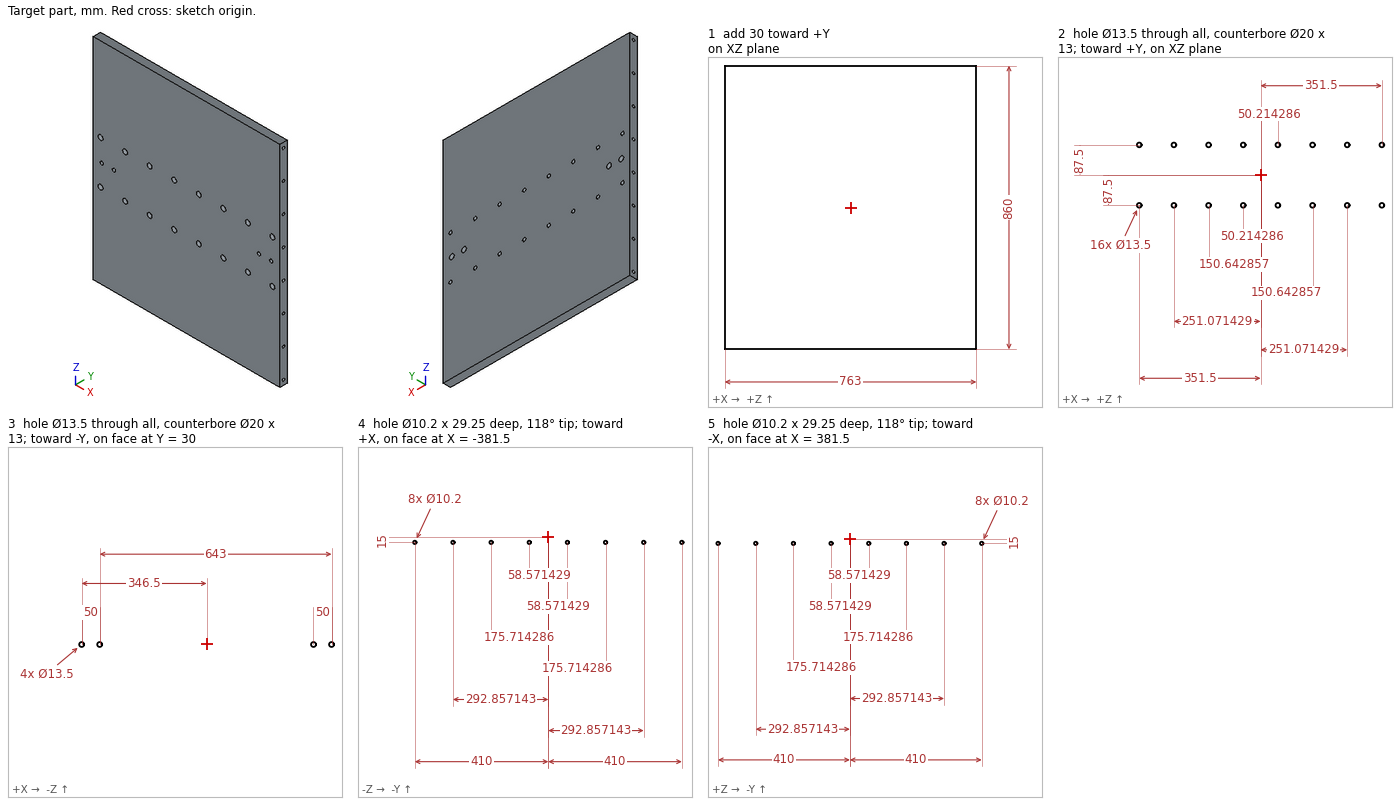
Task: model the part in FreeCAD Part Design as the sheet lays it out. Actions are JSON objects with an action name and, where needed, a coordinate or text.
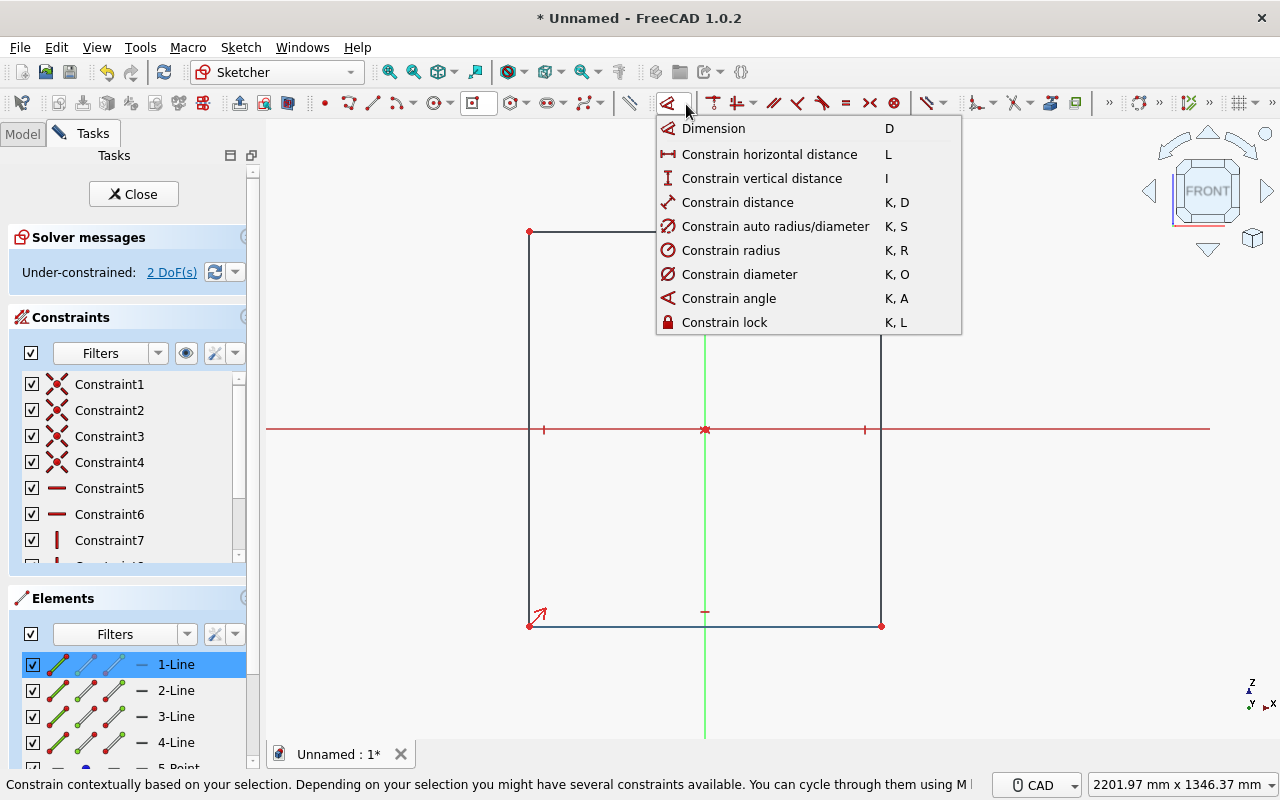
{"action": "left_click", "coordinate": [809, 154]}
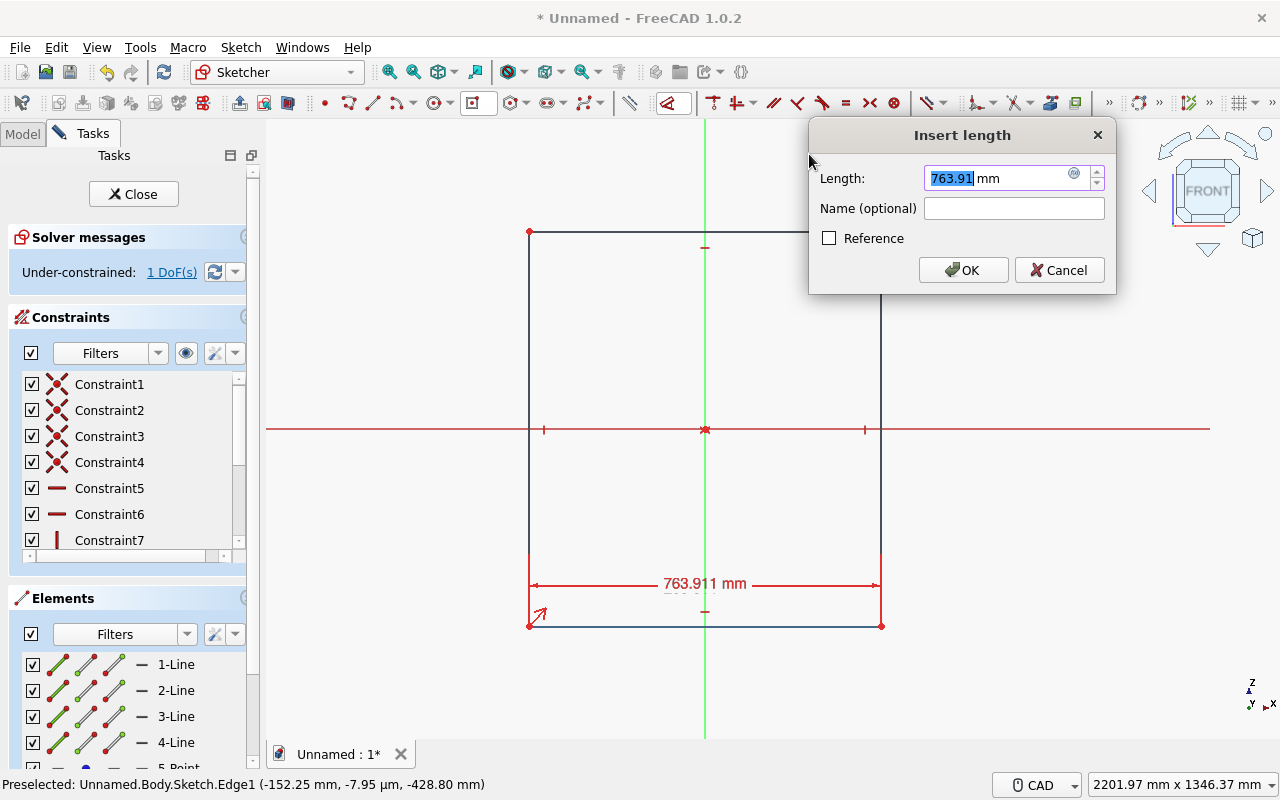
{"action": "type", "text": "763"}
{"action": "key", "text": "Return"}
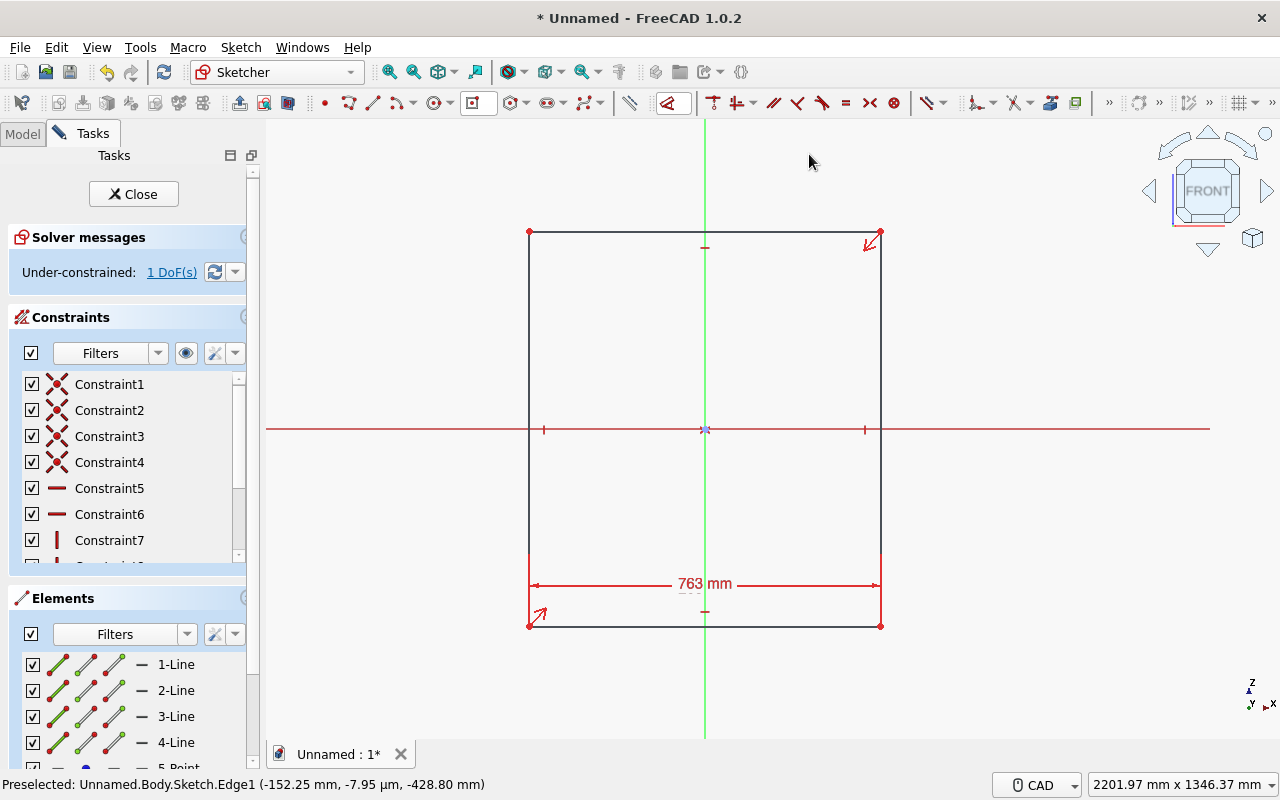
{"action": "left_click", "coordinate": [881, 508]}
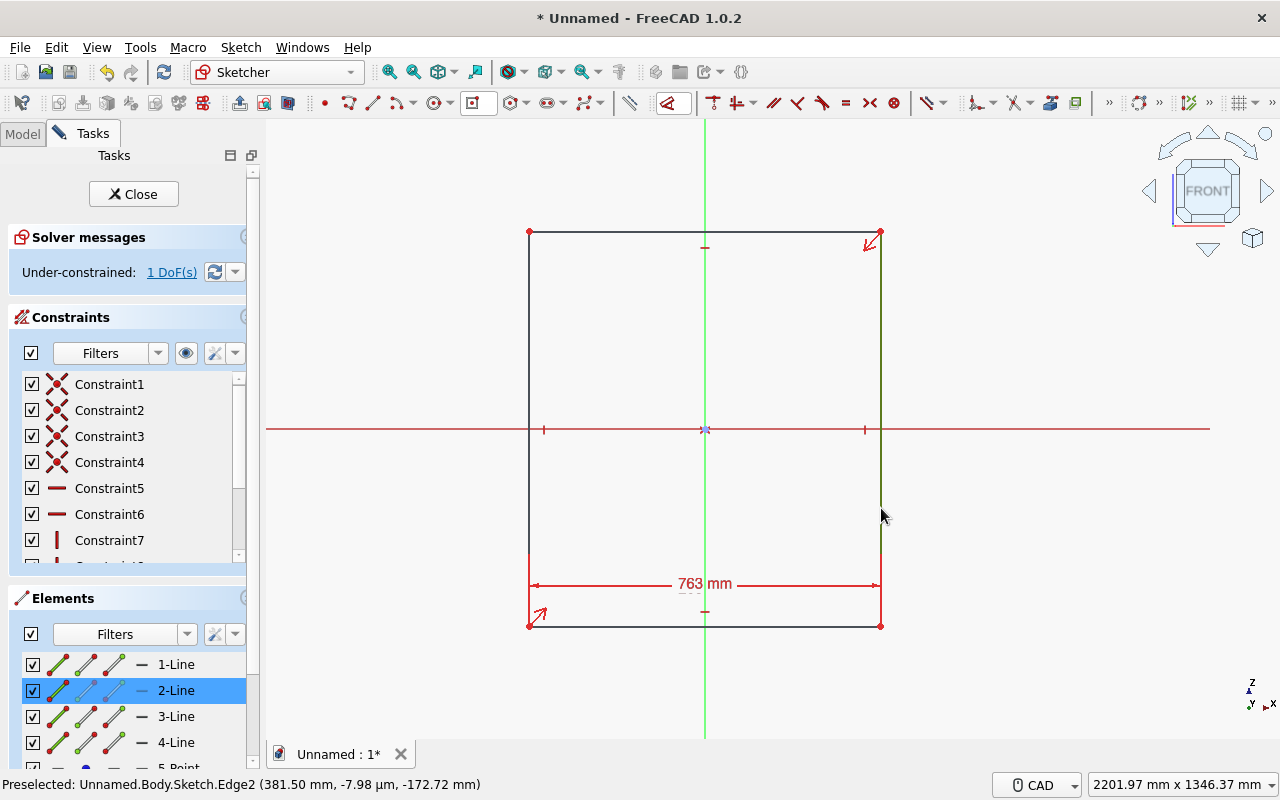
{"action": "left_click", "coordinate": [686, 104]}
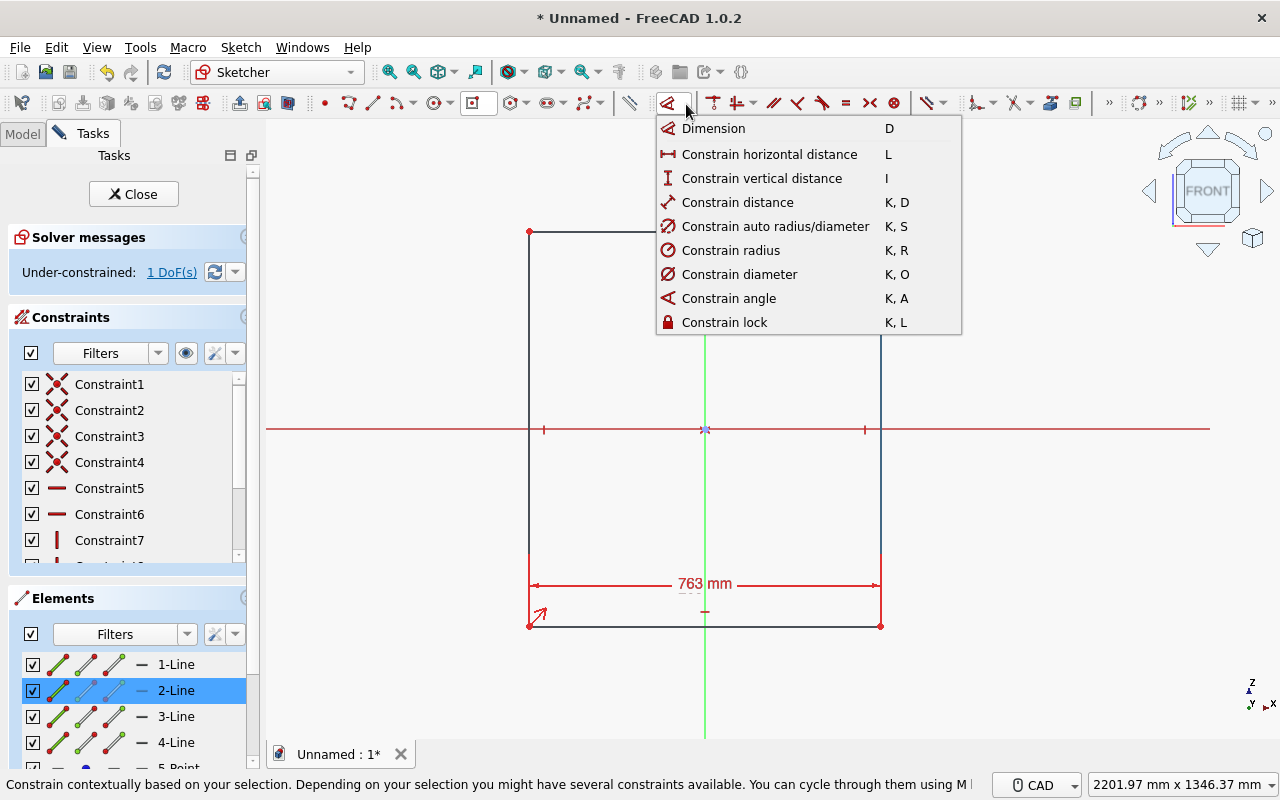
{"action": "left_click", "coordinate": [809, 178]}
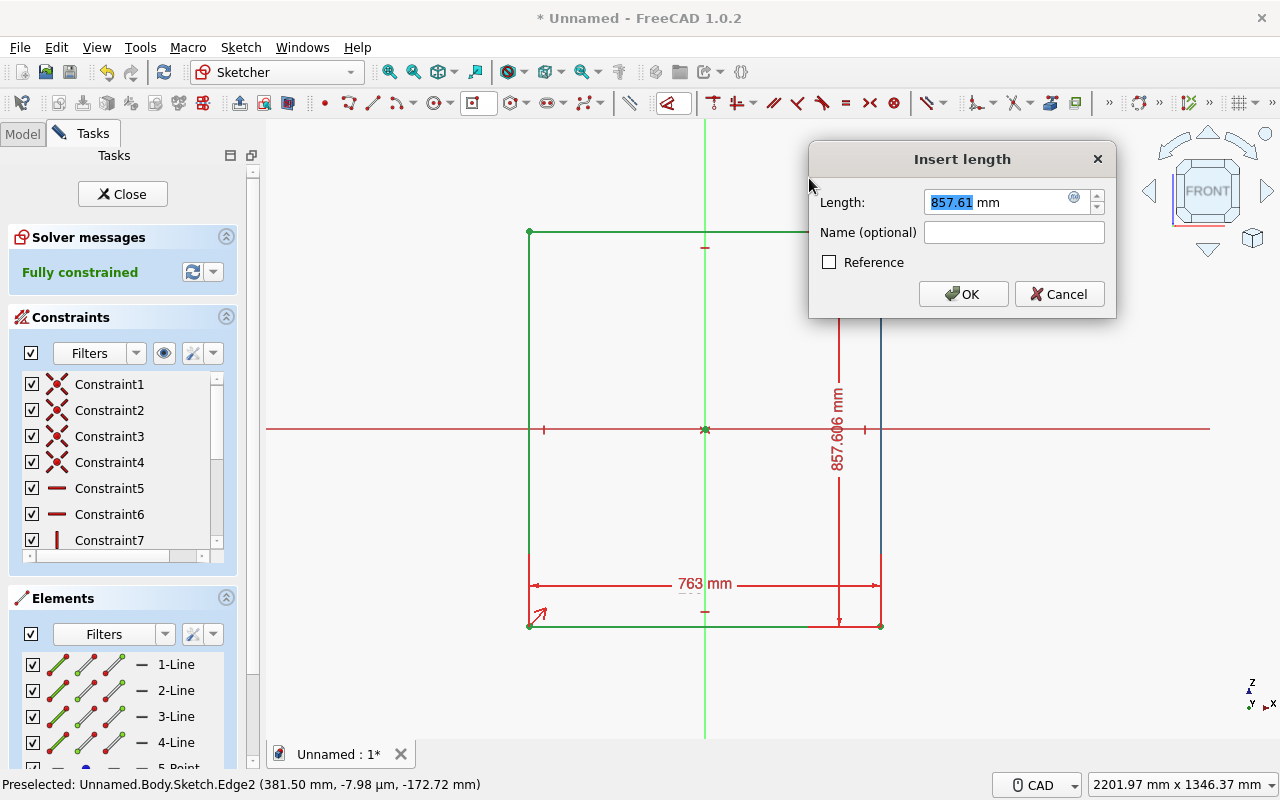
{"action": "type", "text": "860"}
{"action": "key", "text": "Return"}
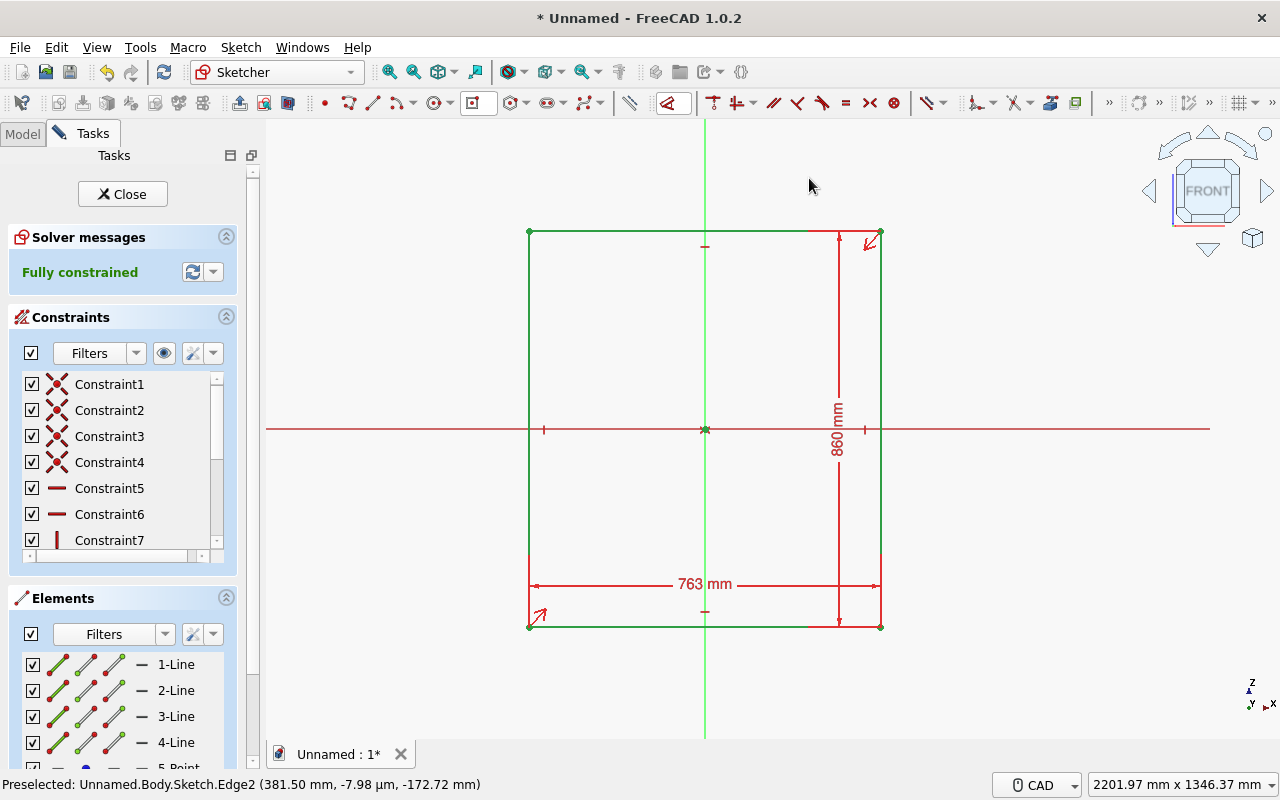
{"action": "left_click", "coordinate": [123, 194]}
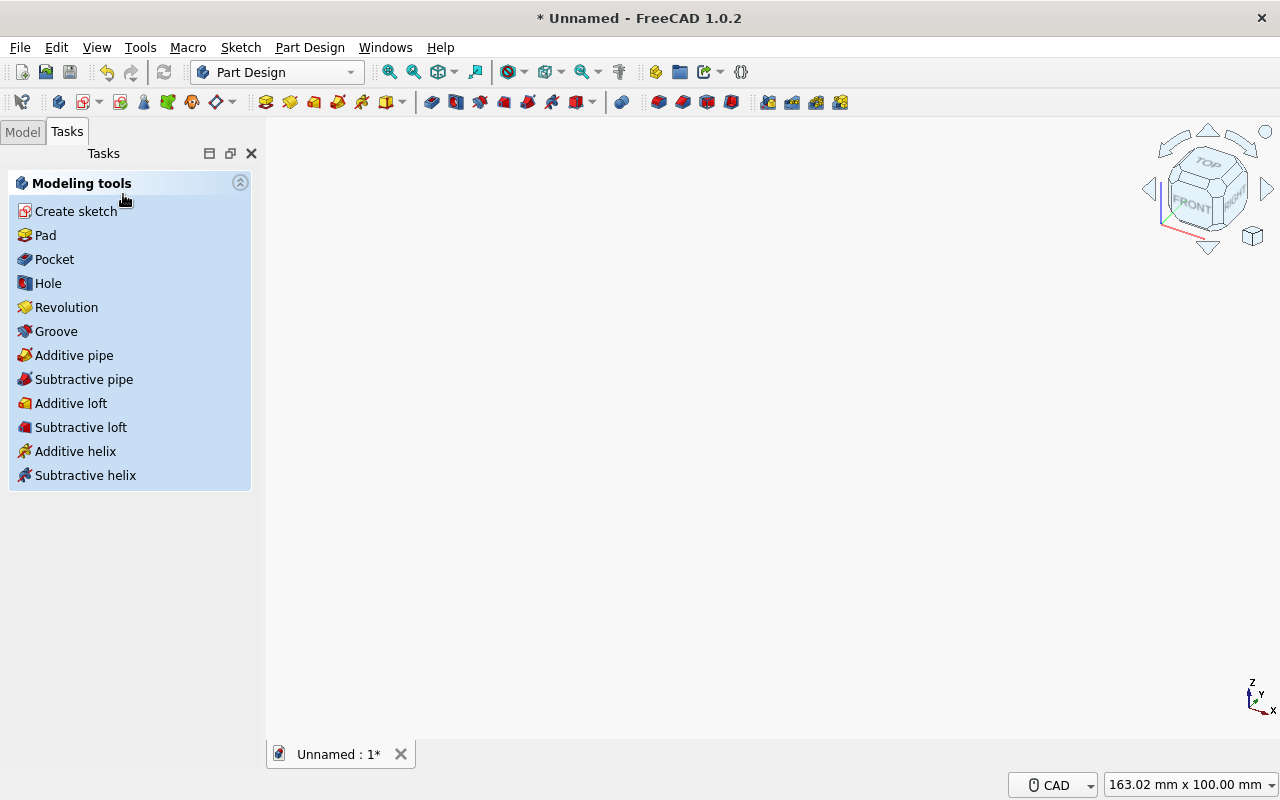
{"action": "left_click", "coordinate": [266, 102]}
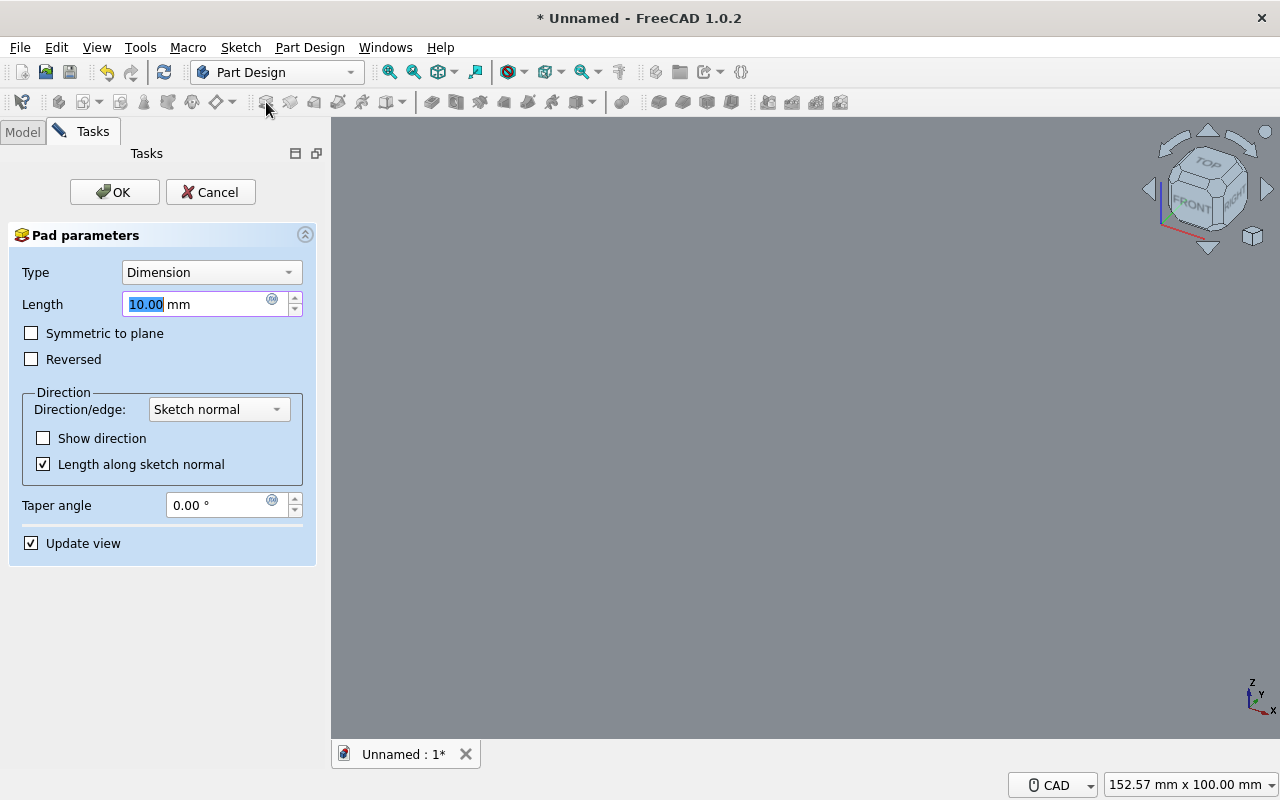
{"action": "type", "text": "30"}
{"action": "key", "text": "Tab"}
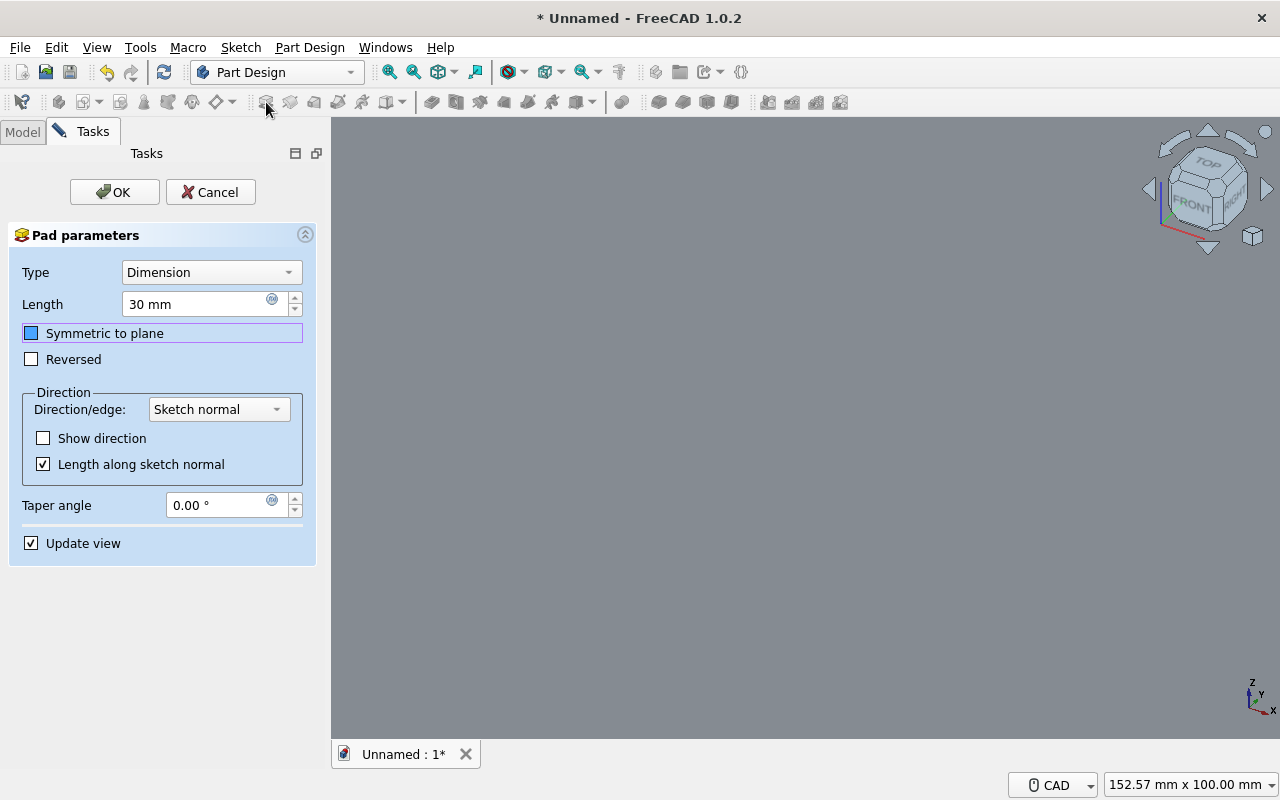
{"action": "left_click", "coordinate": [30, 359]}